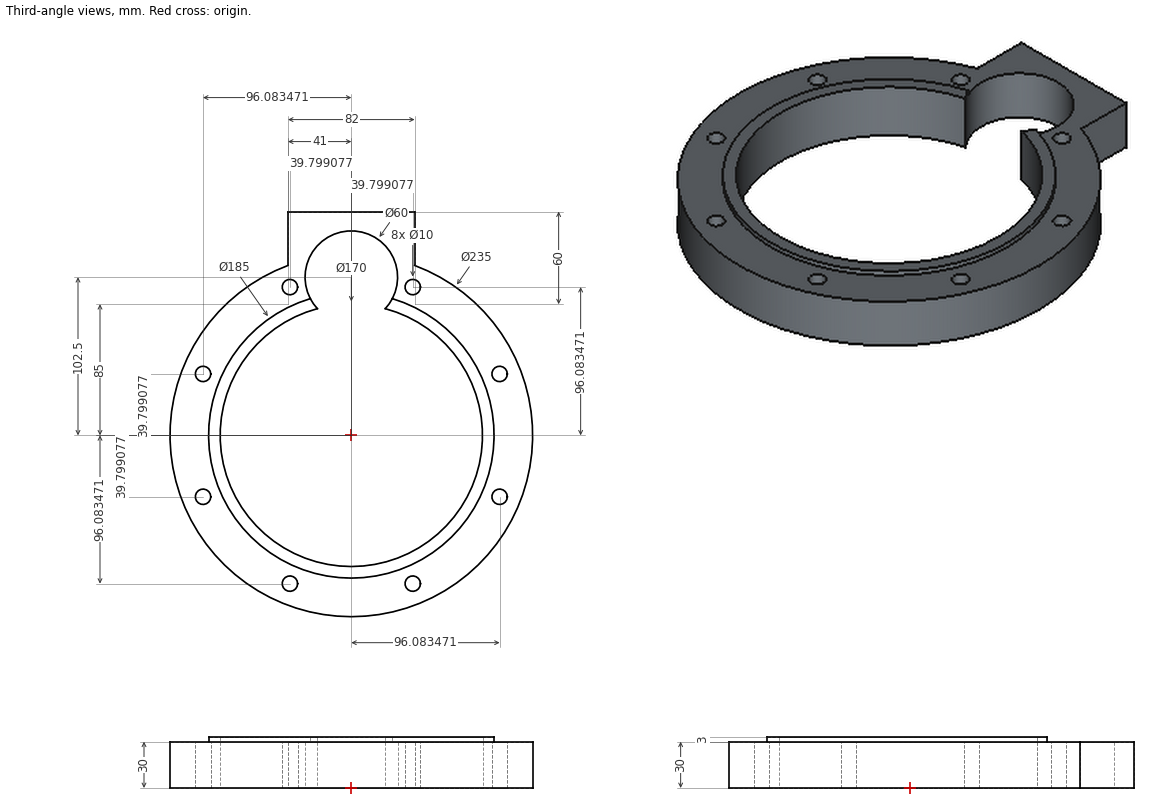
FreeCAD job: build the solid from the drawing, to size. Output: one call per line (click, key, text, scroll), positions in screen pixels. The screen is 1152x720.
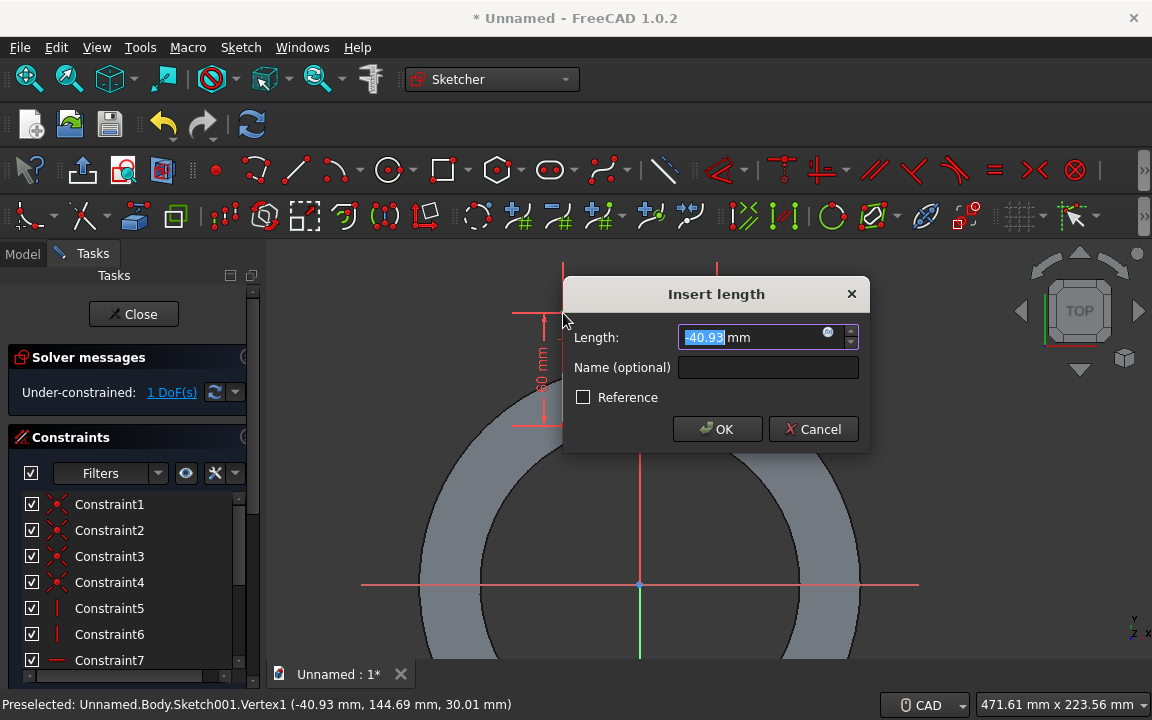
text(-41)
key(Return)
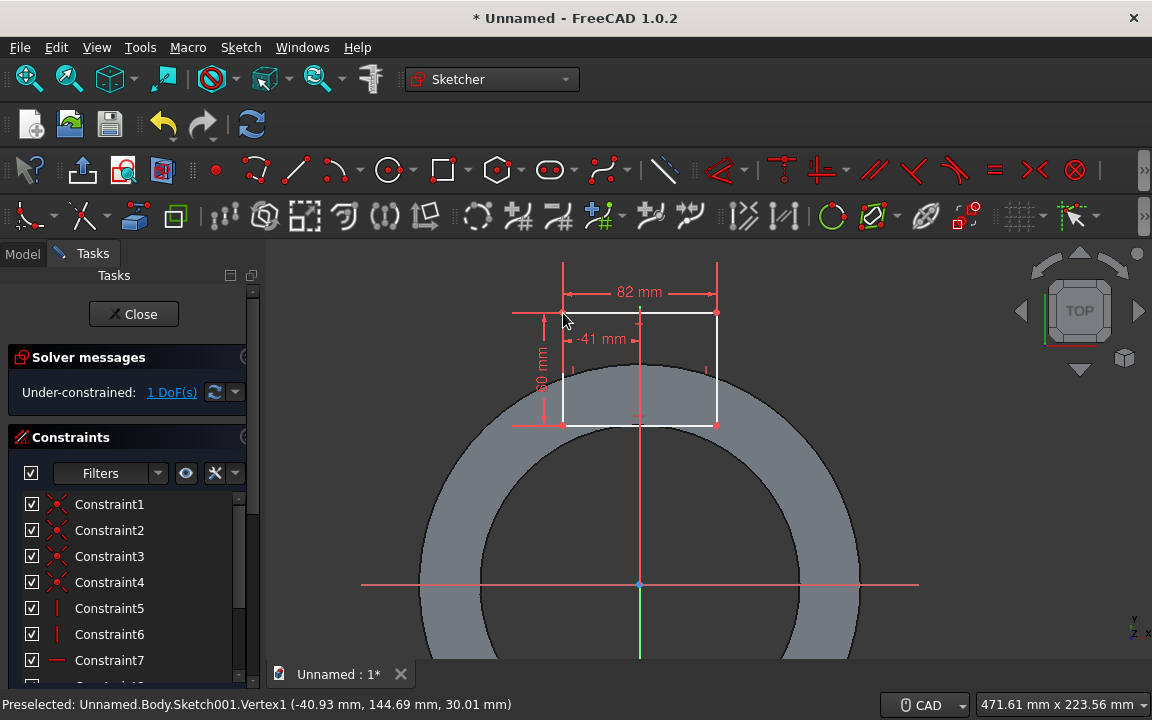
click(563, 426)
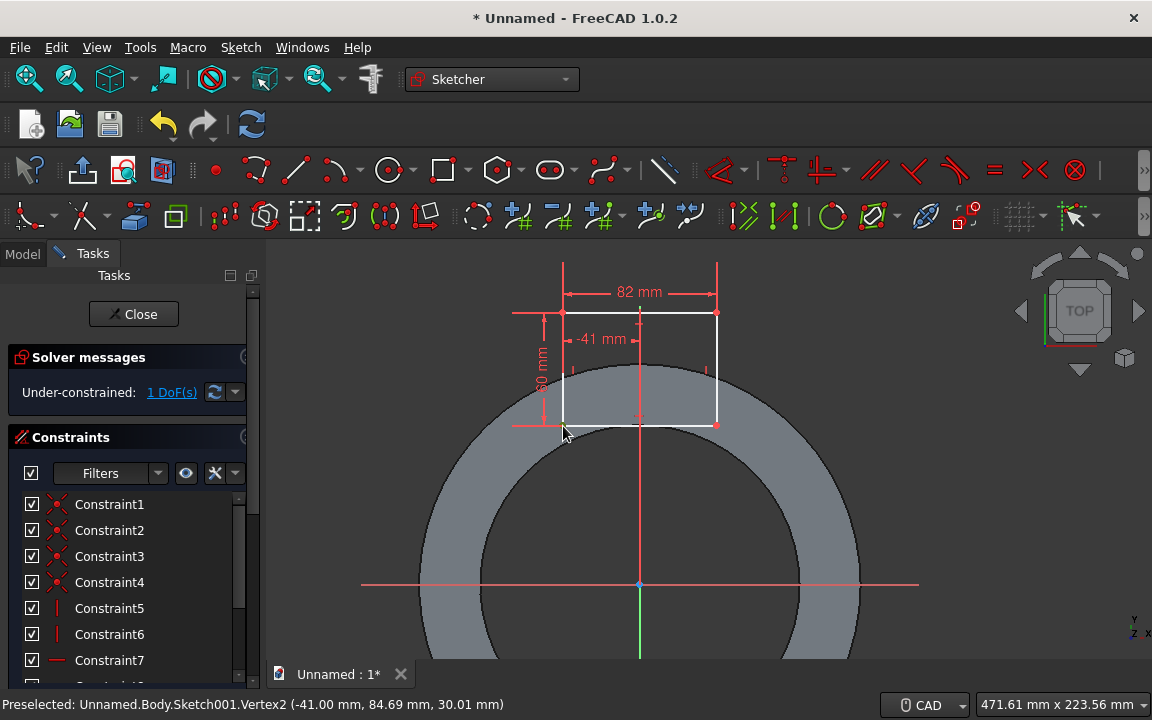
key(i)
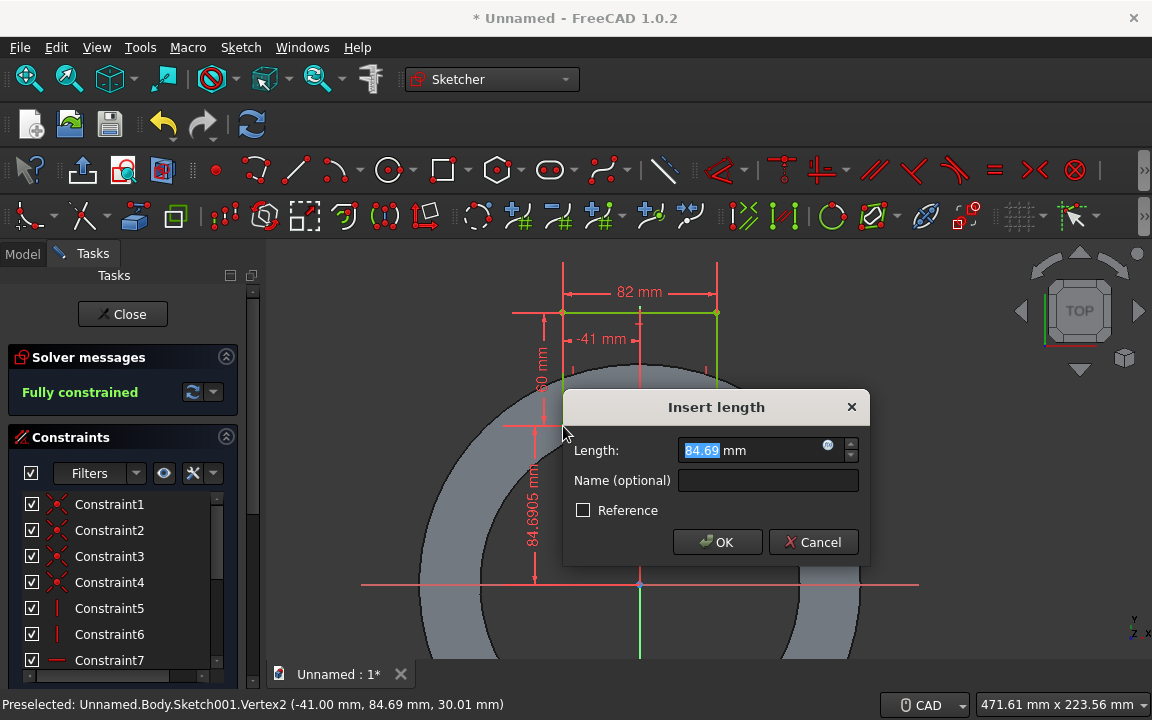
text(85)
key(Return)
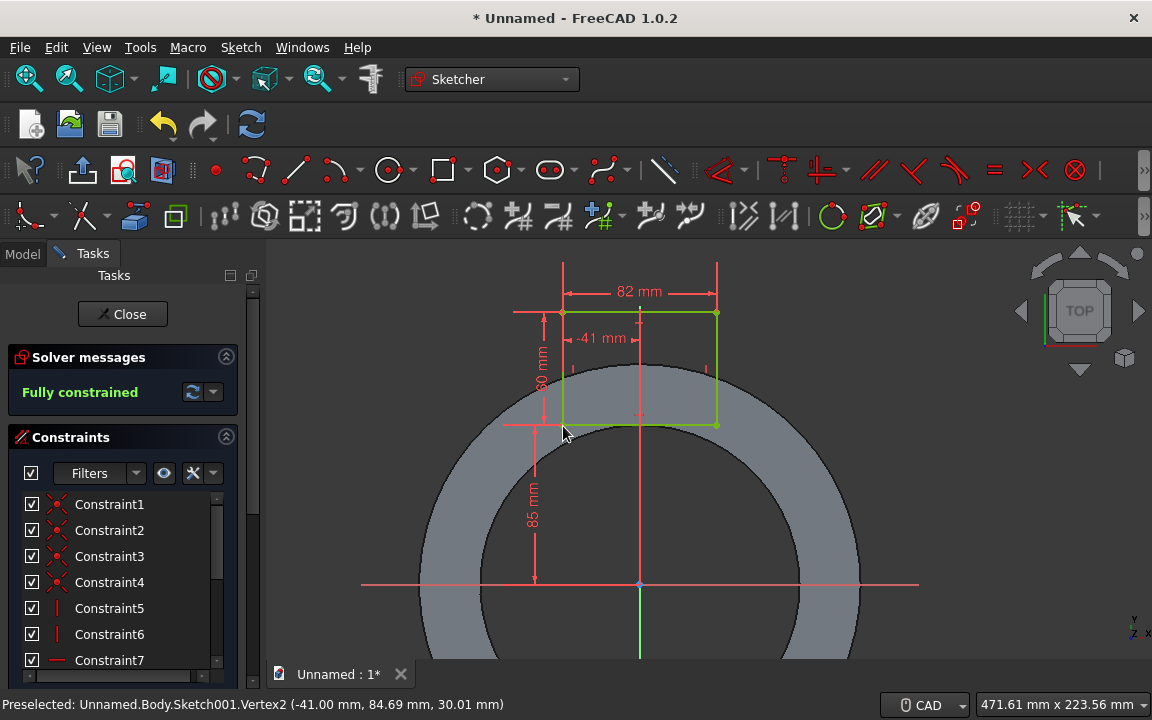
click(123, 314)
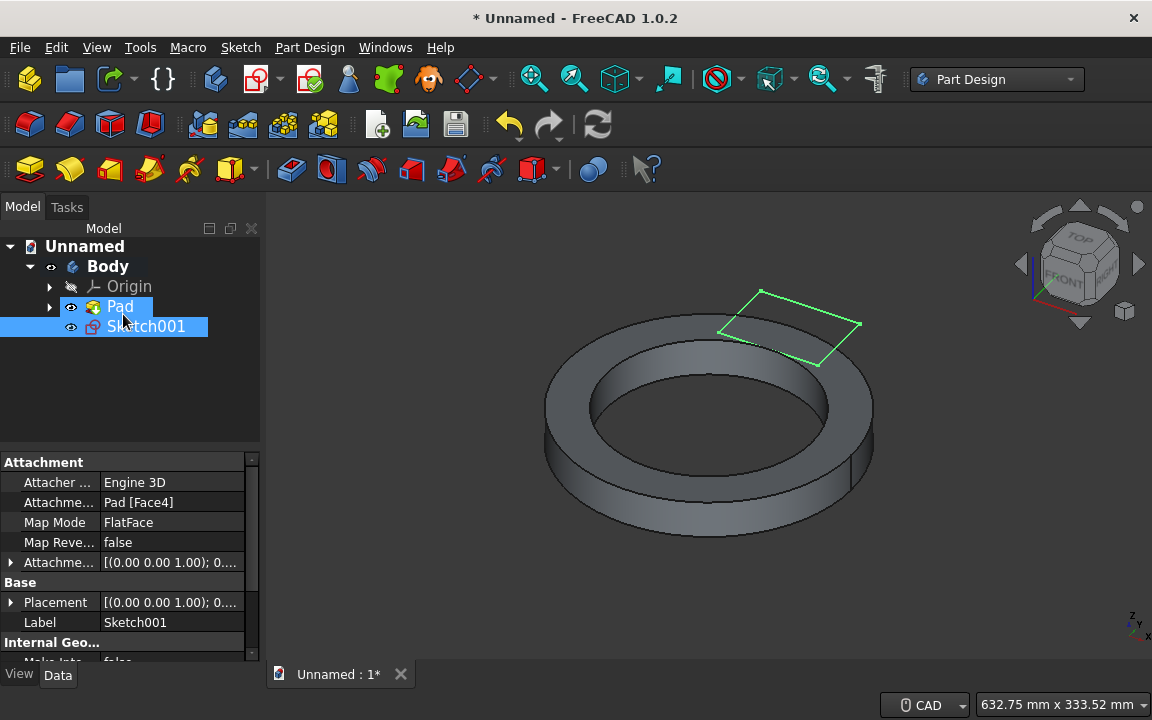
click(30, 170)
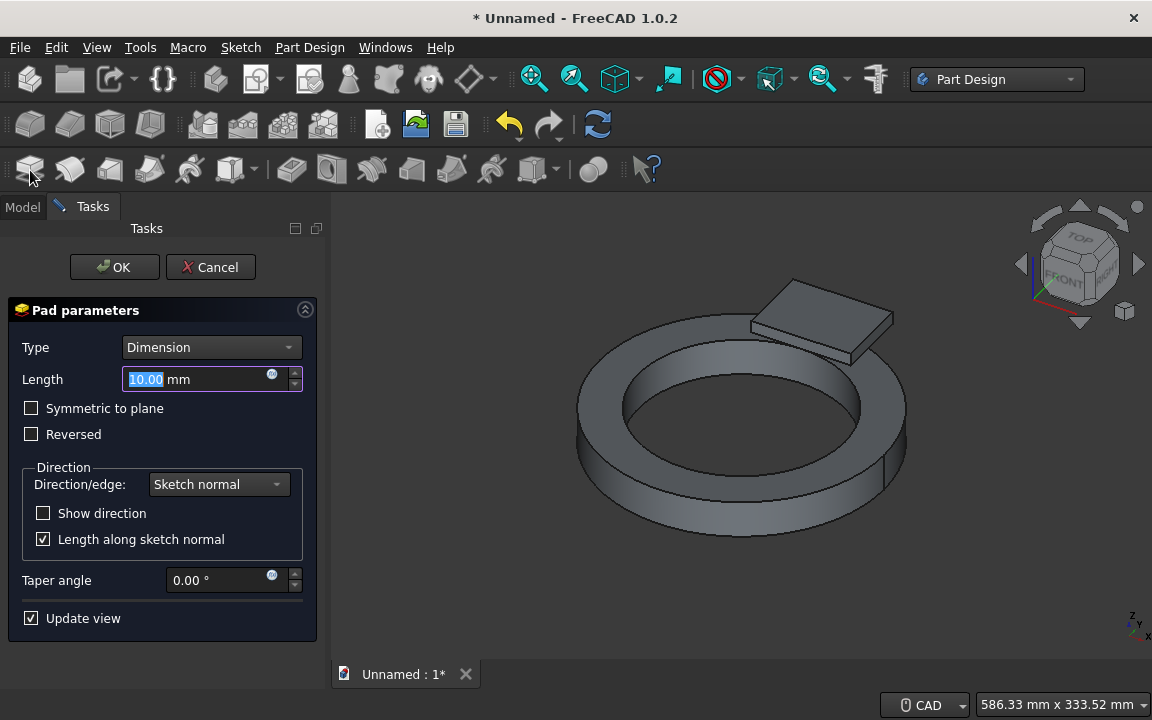
text(30)
key(Tab)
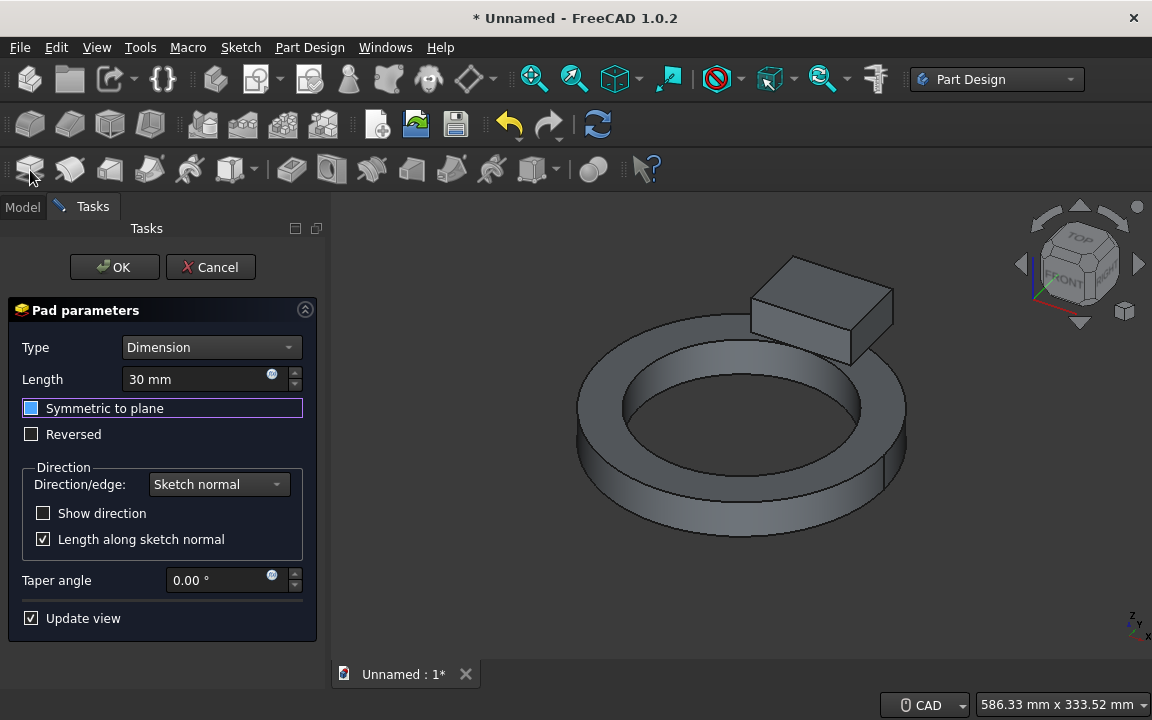
click(30, 434)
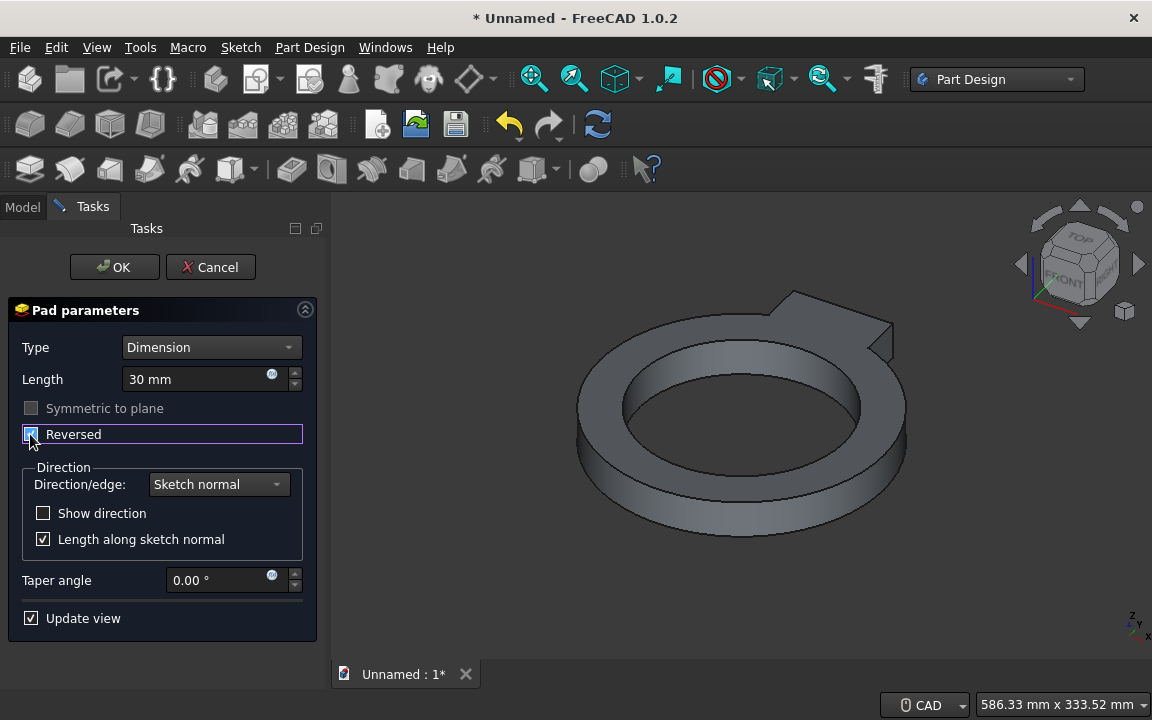
click(115, 267)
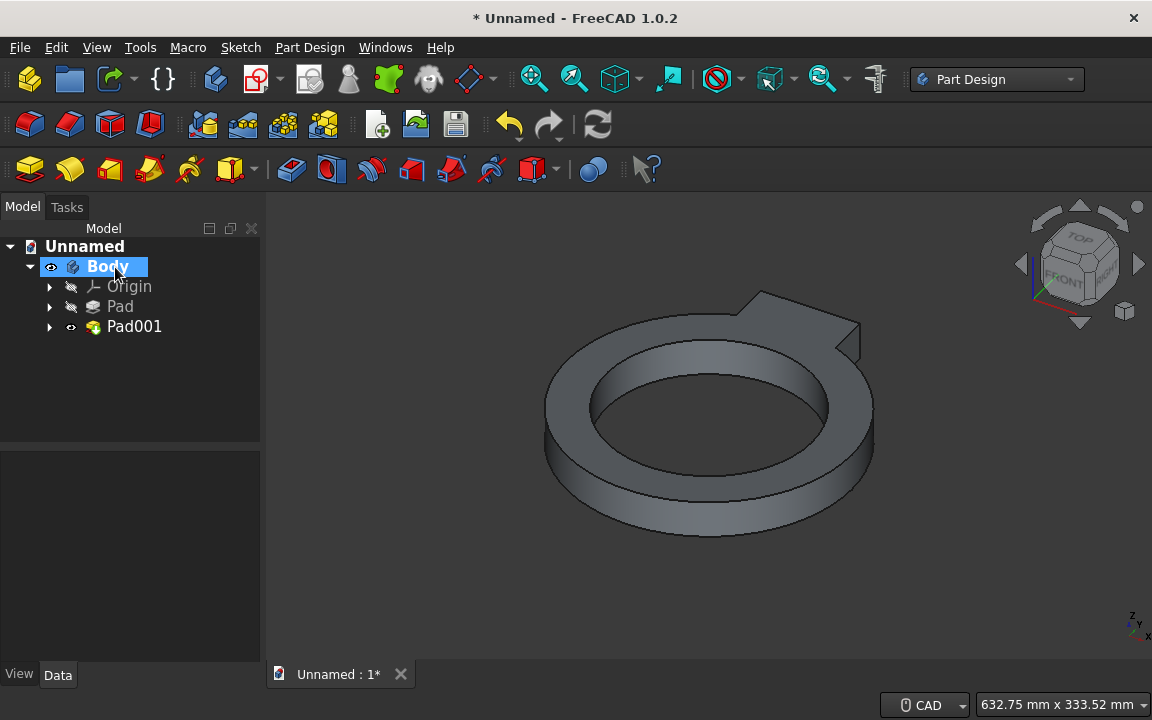
click(256, 80)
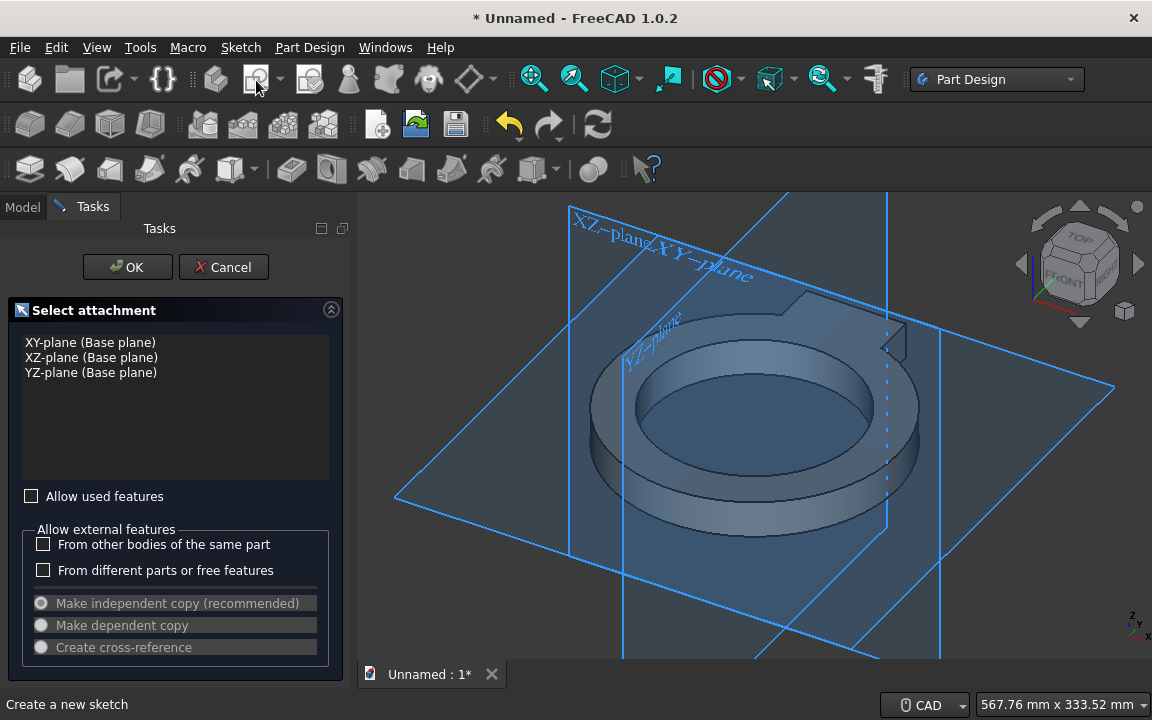
click(82, 342)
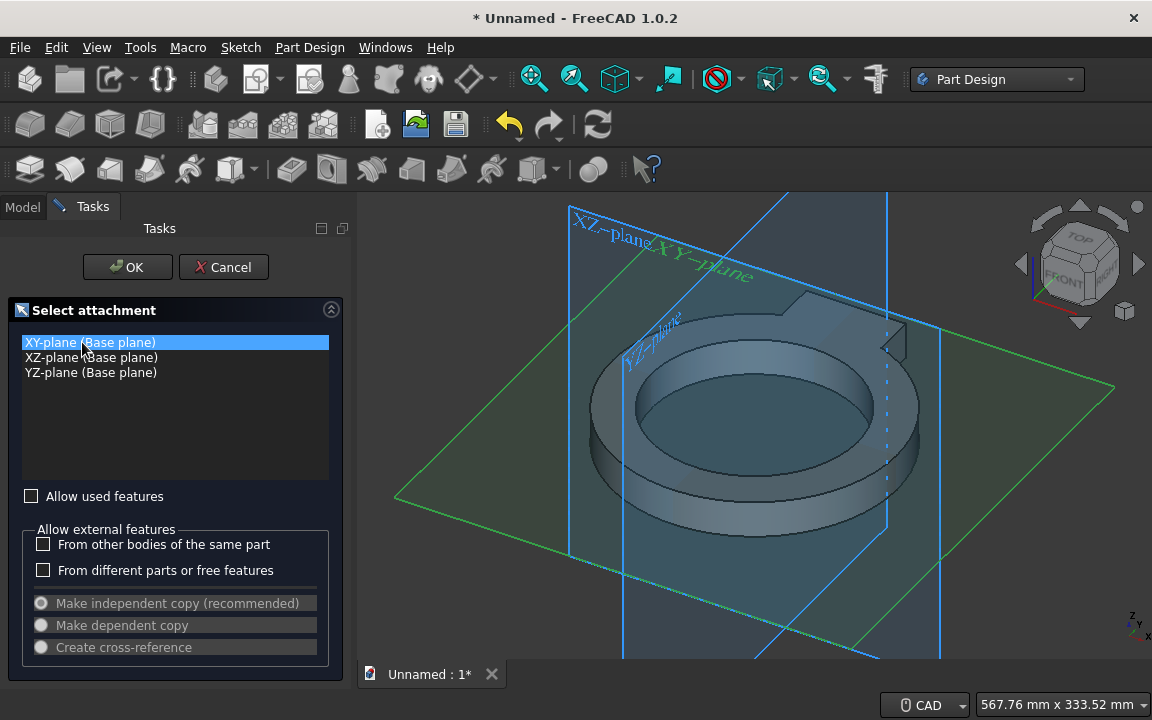
click(128, 267)